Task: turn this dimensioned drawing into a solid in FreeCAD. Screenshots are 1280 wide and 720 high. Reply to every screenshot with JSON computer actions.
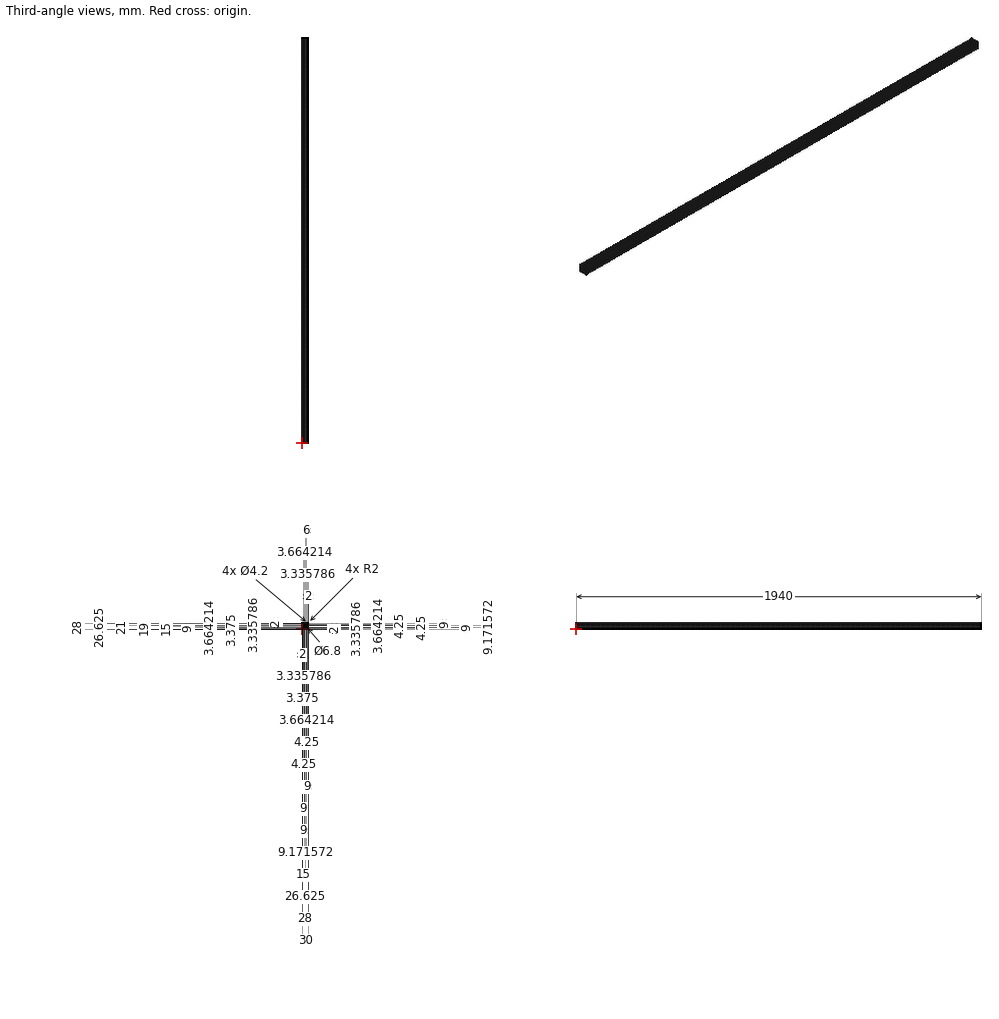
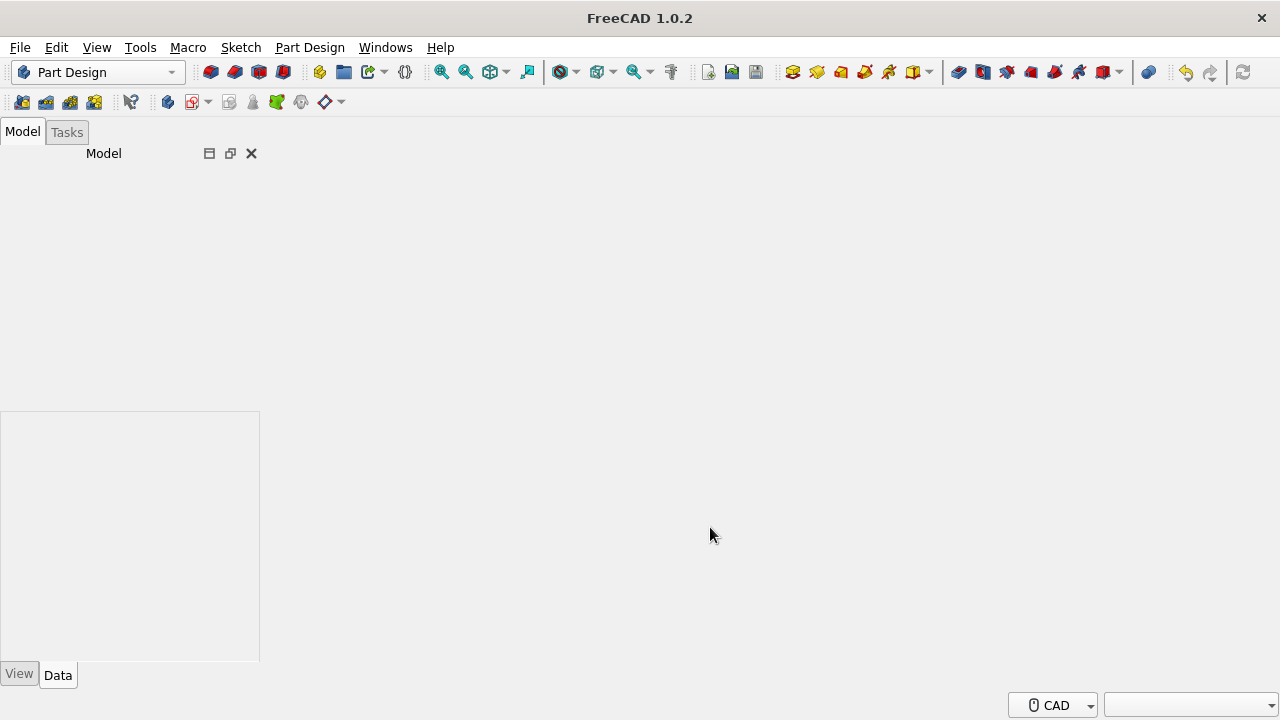
{"action": "left_click", "coordinate": [708, 72]}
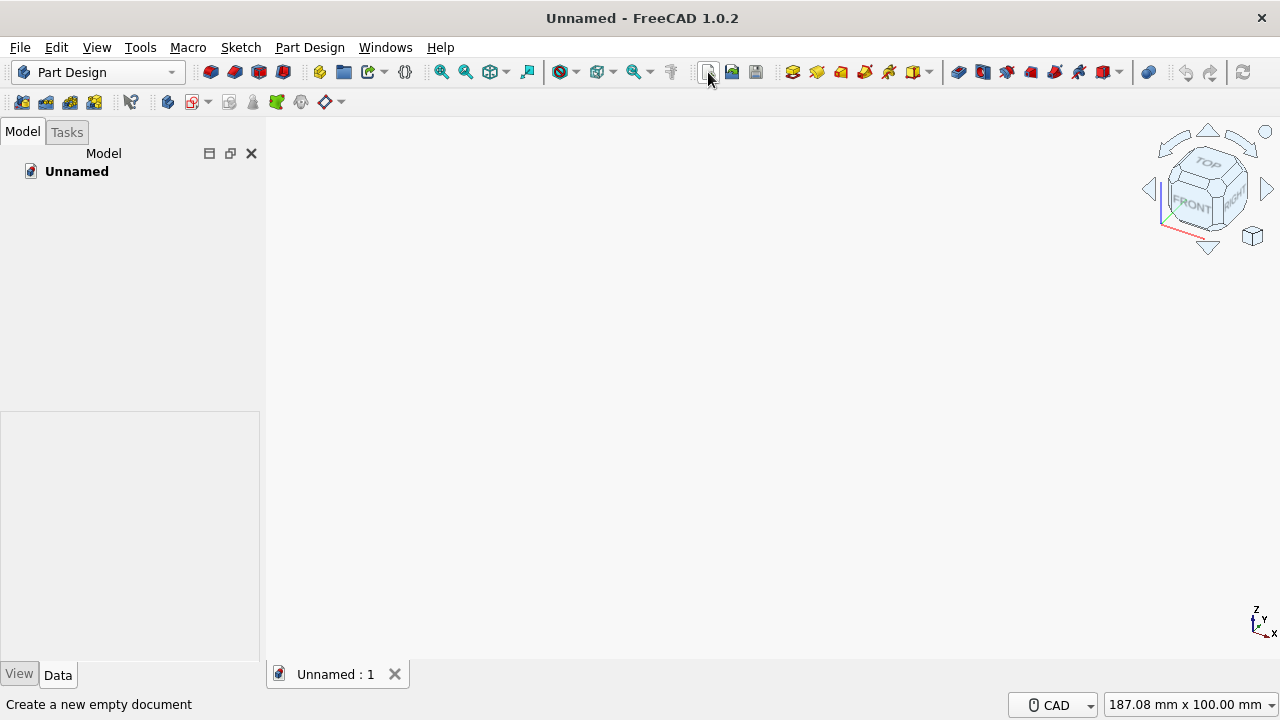
{"action": "left_click", "coordinate": [192, 102]}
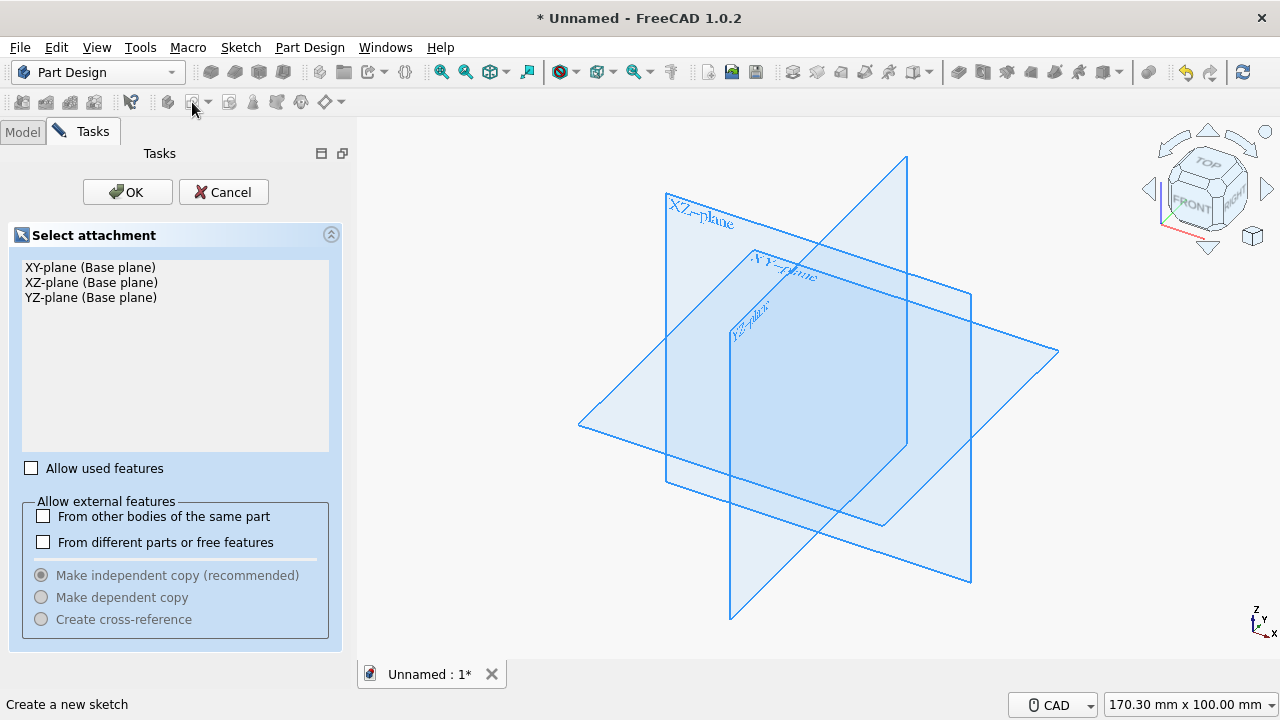
{"action": "left_click", "coordinate": [82, 282]}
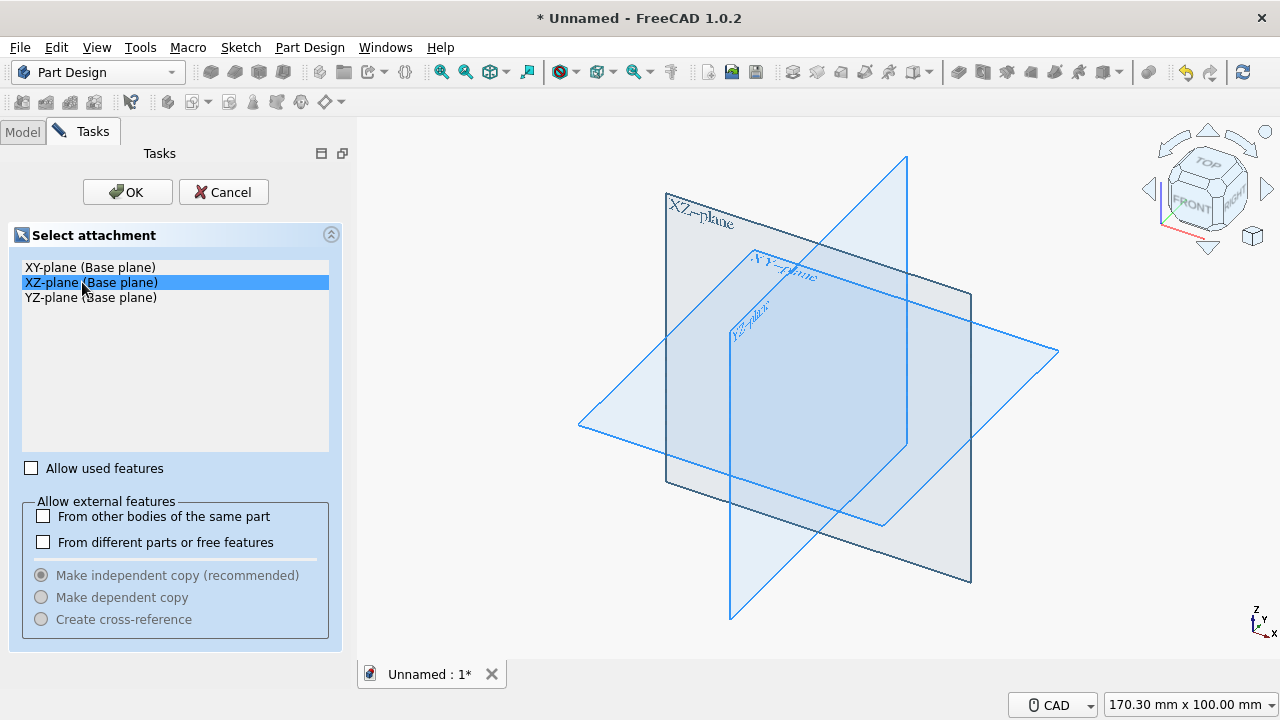
{"action": "left_click", "coordinate": [128, 192]}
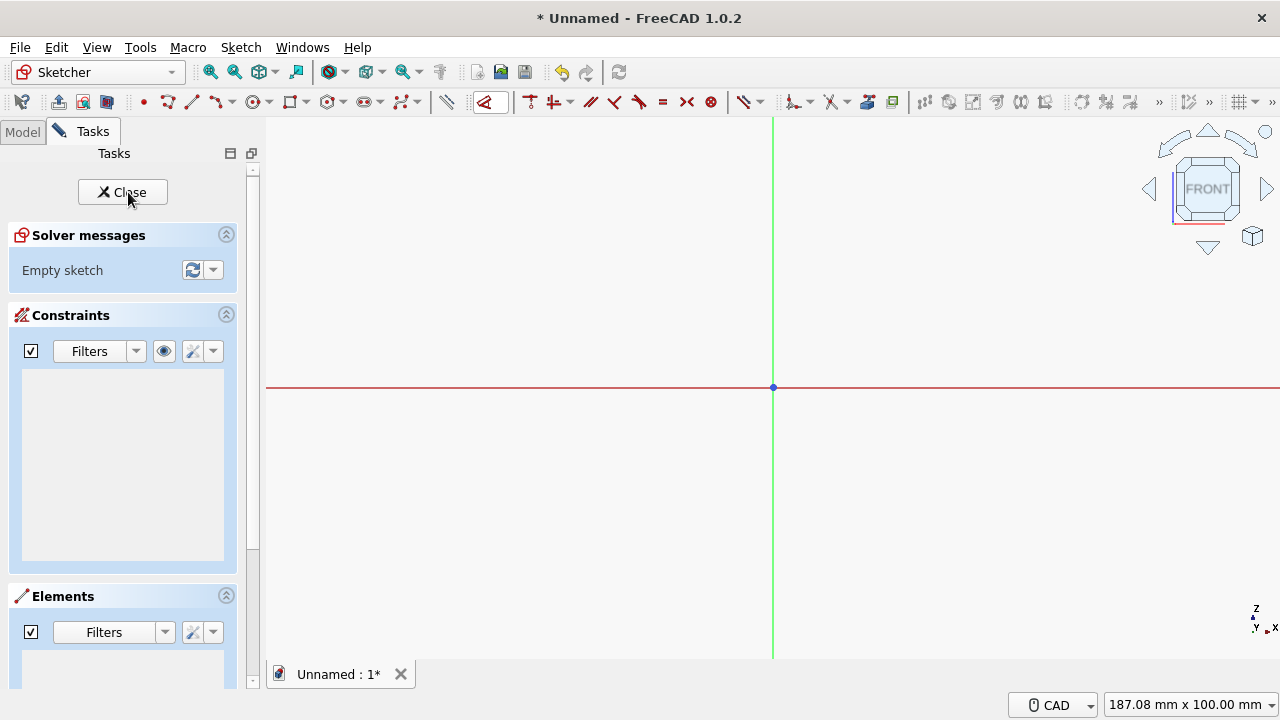
{"action": "scroll", "coordinate": [977, 240], "scroll_direction": "up", "scroll_amount": 4}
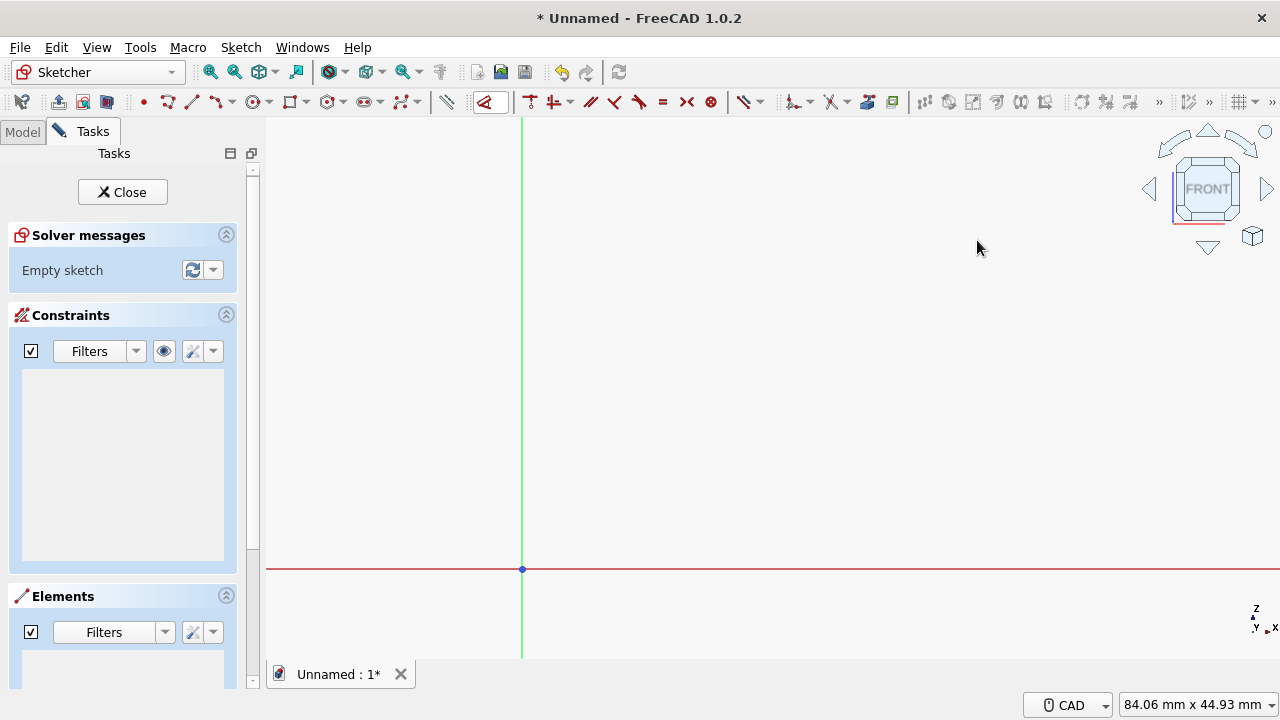
{"action": "key", "text": "g m"}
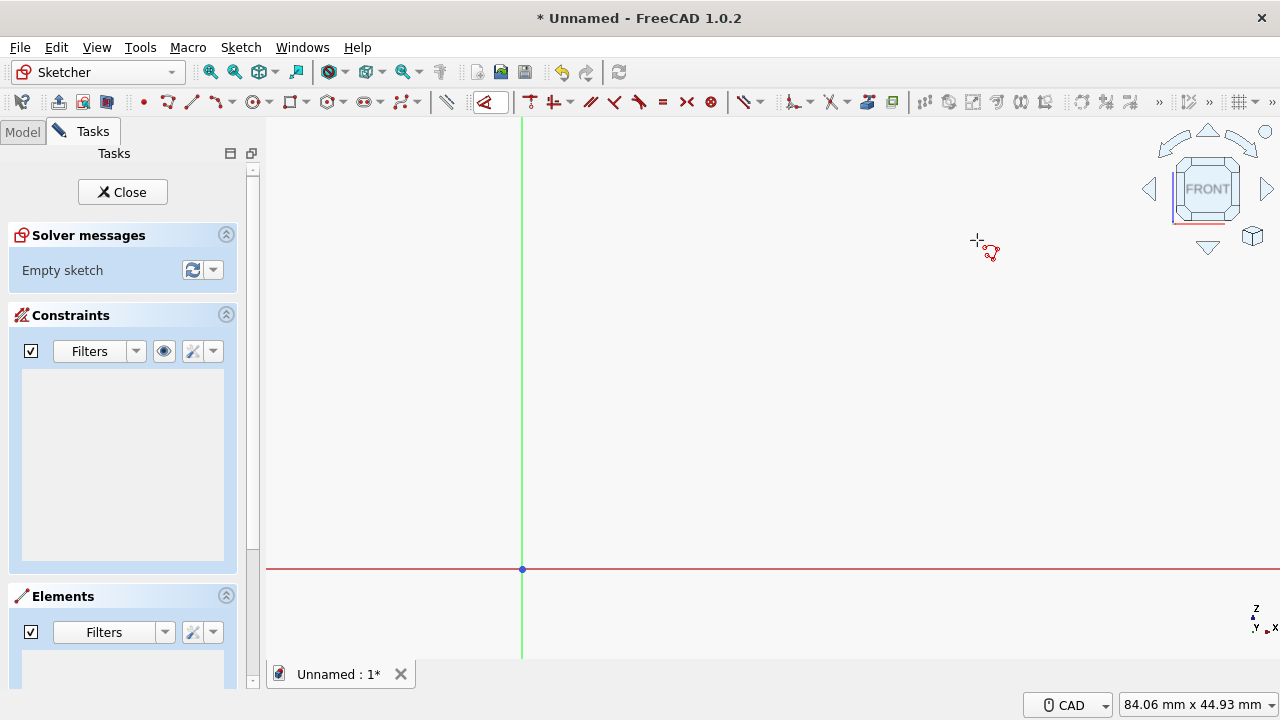
{"action": "left_click", "coordinate": [884, 231]}
{"action": "left_click", "coordinate": [884, 340]}
{"action": "left_click", "coordinate": [860, 340]}
{"action": "left_click", "coordinate": [860, 289]}
{"action": "left_click", "coordinate": [820, 289]}
{"action": "left_click", "coordinate": [775, 333]}
{"action": "left_click", "coordinate": [775, 443]}
{"action": "left_click", "coordinate": [820, 488]}
{"action": "left_click", "coordinate": [860, 488]}
{"action": "left_click", "coordinate": [860, 436]}
{"action": "left_click", "coordinate": [884, 436]}
{"action": "left_click", "coordinate": [884, 545]}
{"action": "right_click", "coordinate": [884, 545]}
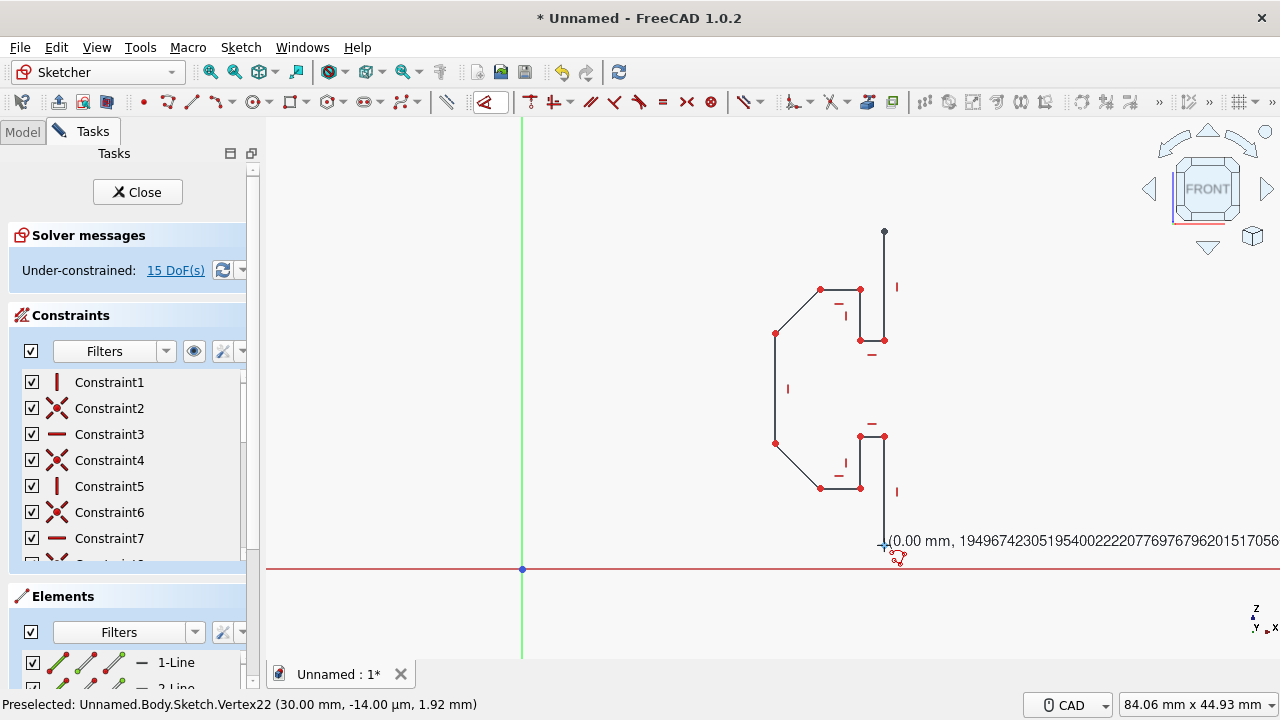
{"action": "left_click", "coordinate": [860, 569]}
{"action": "left_click", "coordinate": [751, 560]}
{"action": "left_click", "coordinate": [751, 545]}
{"action": "left_click", "coordinate": [803, 545]}
{"action": "left_click", "coordinate": [803, 505]}
{"action": "left_click", "coordinate": [758, 461]}
{"action": "left_click", "coordinate": [648, 461]}
{"action": "left_click", "coordinate": [604, 505]}
{"action": "left_click", "coordinate": [604, 545]}
{"action": "left_click", "coordinate": [655, 545]}
{"action": "left_click", "coordinate": [655, 569]}
{"action": "left_click", "coordinate": [546, 560]}
{"action": "right_click", "coordinate": [546, 560]}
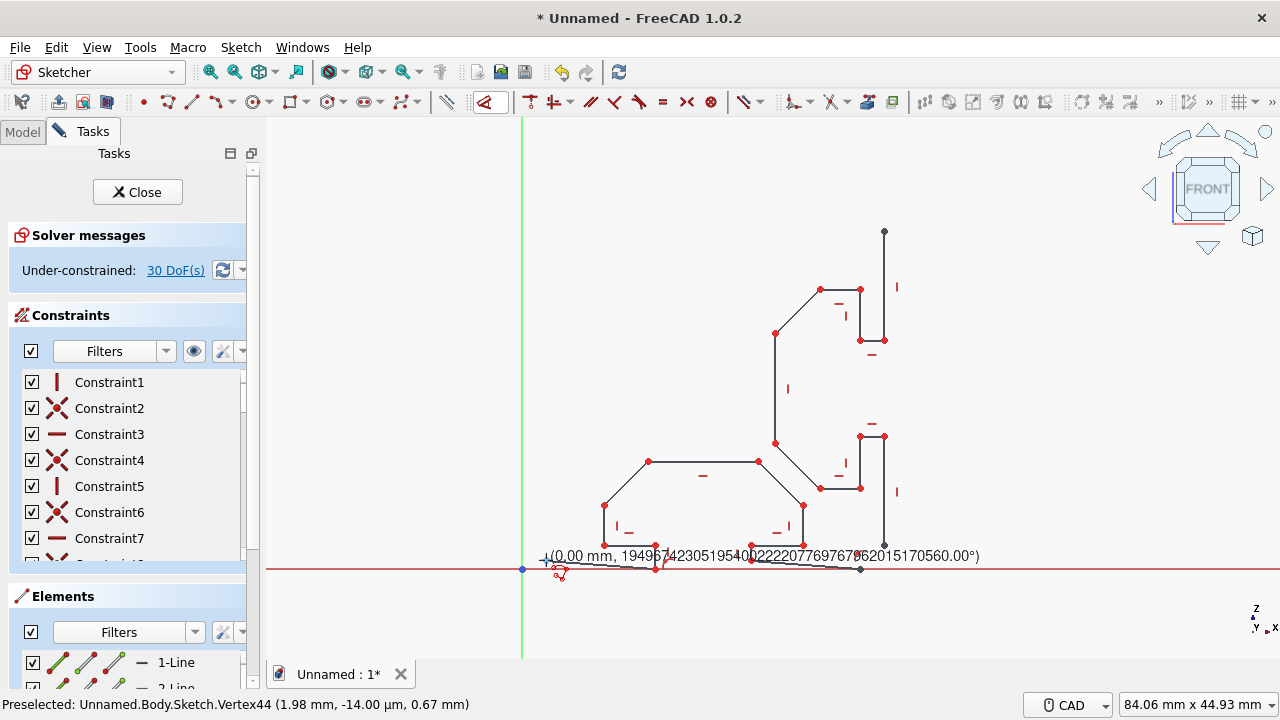
{"action": "left_click", "coordinate": [522, 545]}
{"action": "left_click", "coordinate": [531, 436]}
{"action": "left_click", "coordinate": [546, 436]}
{"action": "left_click", "coordinate": [546, 488]}
{"action": "left_click", "coordinate": [586, 488]}
{"action": "left_click", "coordinate": [631, 443]}
{"action": "left_click", "coordinate": [631, 333]}
{"action": "left_click", "coordinate": [586, 289]}
{"action": "left_click", "coordinate": [546, 289]}
{"action": "left_click", "coordinate": [546, 340]}
{"action": "left_click", "coordinate": [522, 340]}
{"action": "left_click", "coordinate": [531, 231]}
{"action": "right_click", "coordinate": [531, 231]}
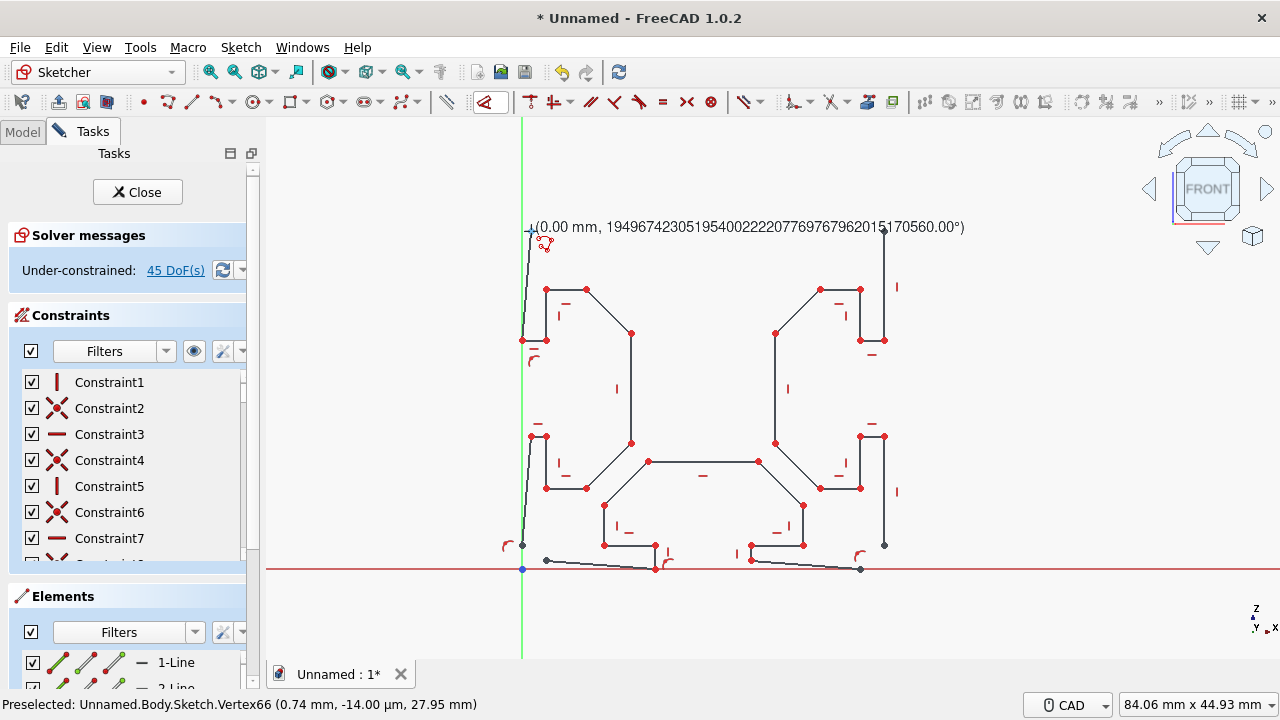
{"action": "left_click", "coordinate": [546, 207]}
{"action": "left_click", "coordinate": [655, 207]}
{"action": "left_click", "coordinate": [655, 231]}
{"action": "left_click", "coordinate": [604, 231]}
{"action": "left_click", "coordinate": [604, 272]}
{"action": "left_click", "coordinate": [648, 316]}
{"action": "left_click", "coordinate": [758, 316]}
{"action": "left_click", "coordinate": [803, 272]}
{"action": "left_click", "coordinate": [803, 231]}
{"action": "left_click", "coordinate": [751, 231]}
{"action": "left_click", "coordinate": [751, 207]}
{"action": "left_click", "coordinate": [860, 207]}
{"action": "right_click", "coordinate": [860, 207]}